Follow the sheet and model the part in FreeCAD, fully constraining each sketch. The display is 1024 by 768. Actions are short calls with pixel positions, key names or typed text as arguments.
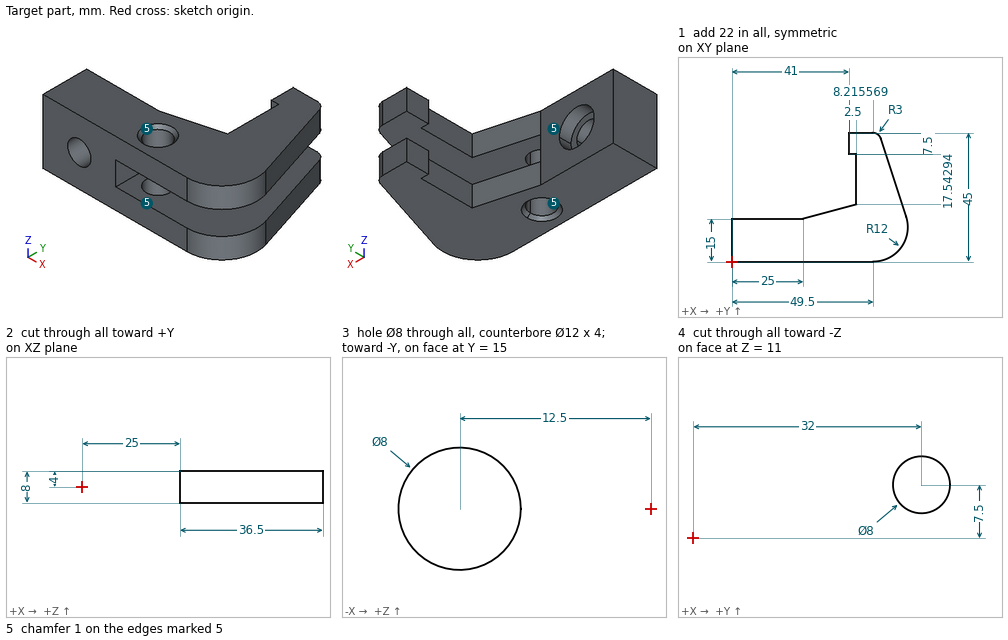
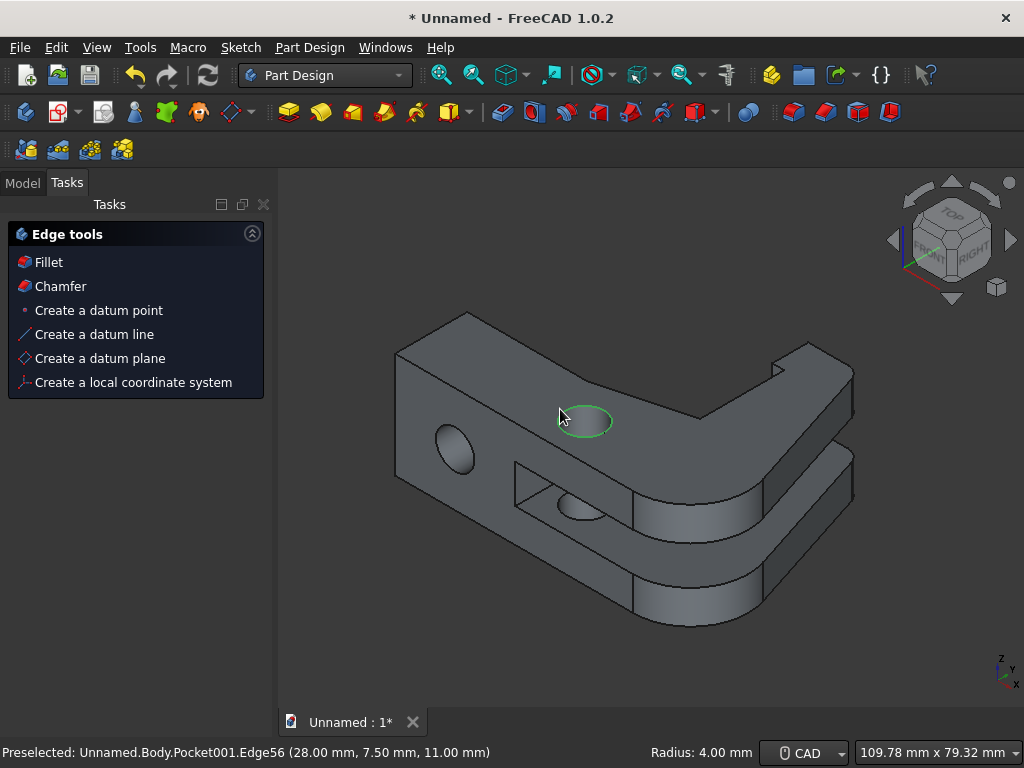
key(2)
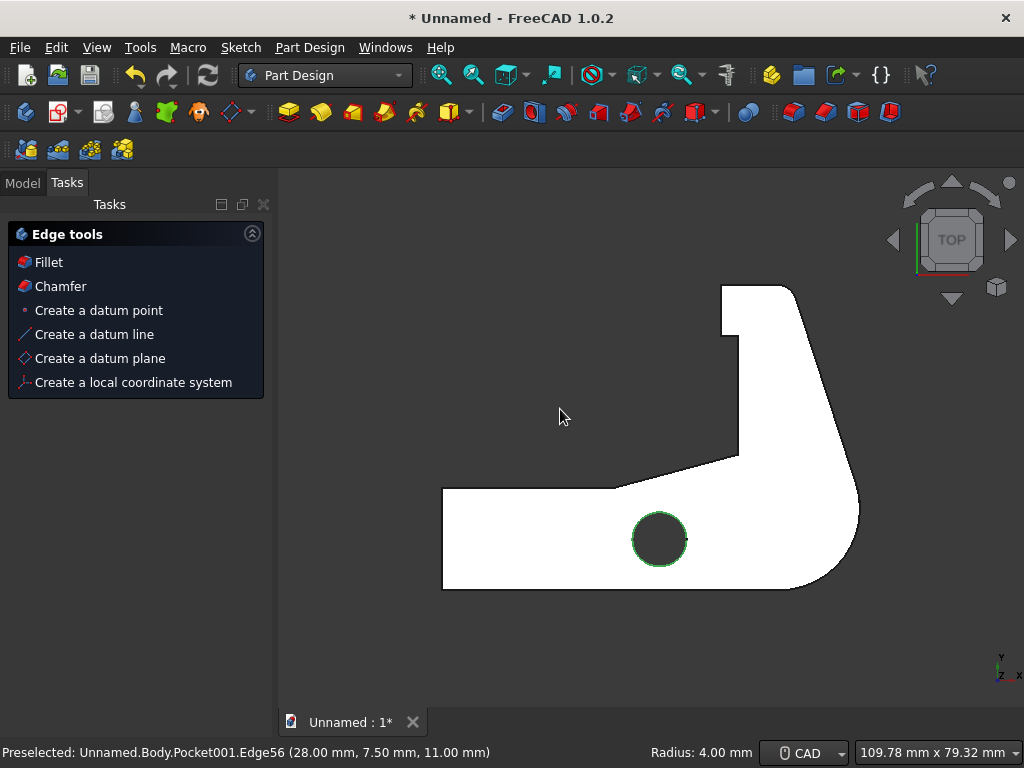
key(0)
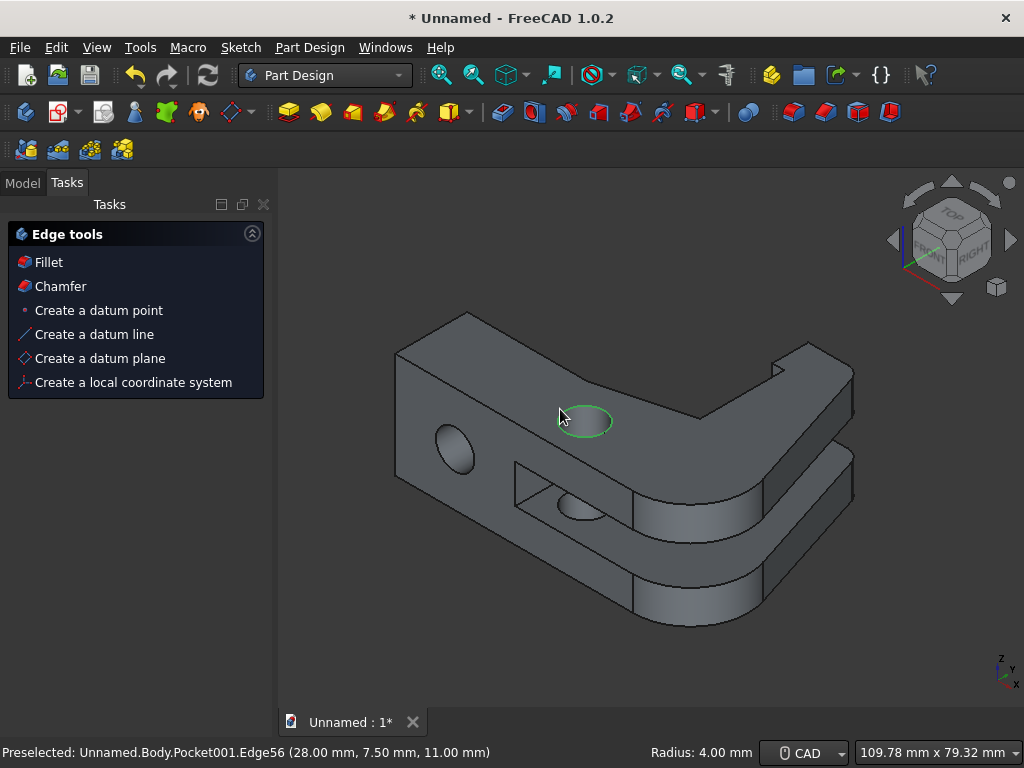
key(1)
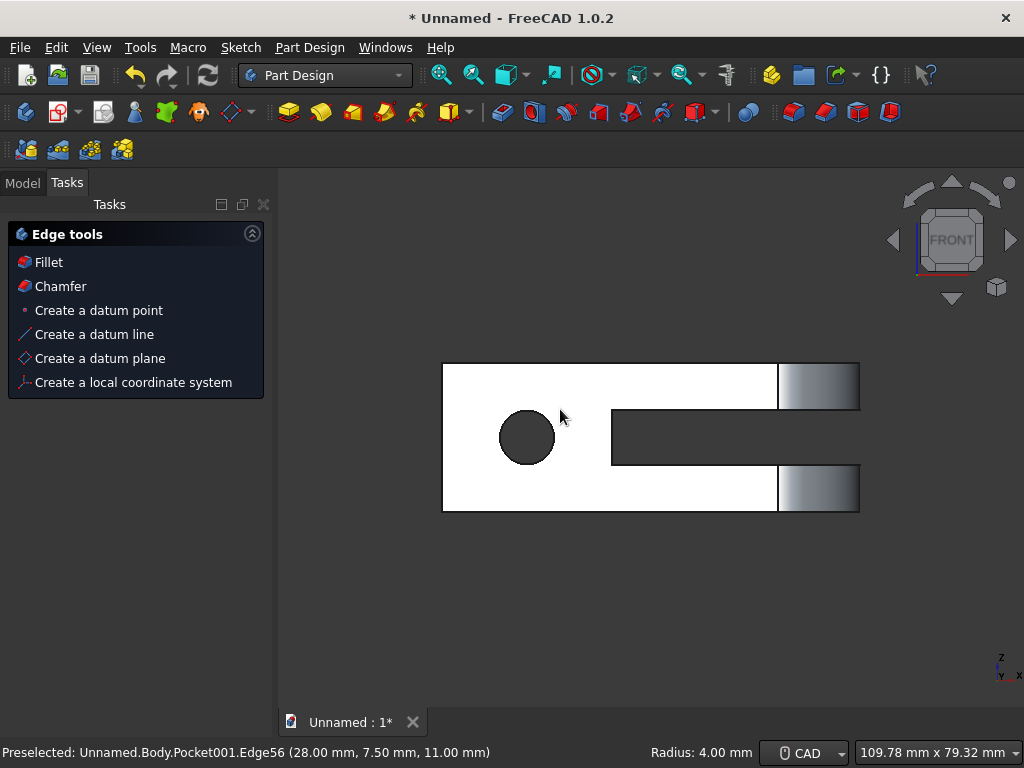
key(3)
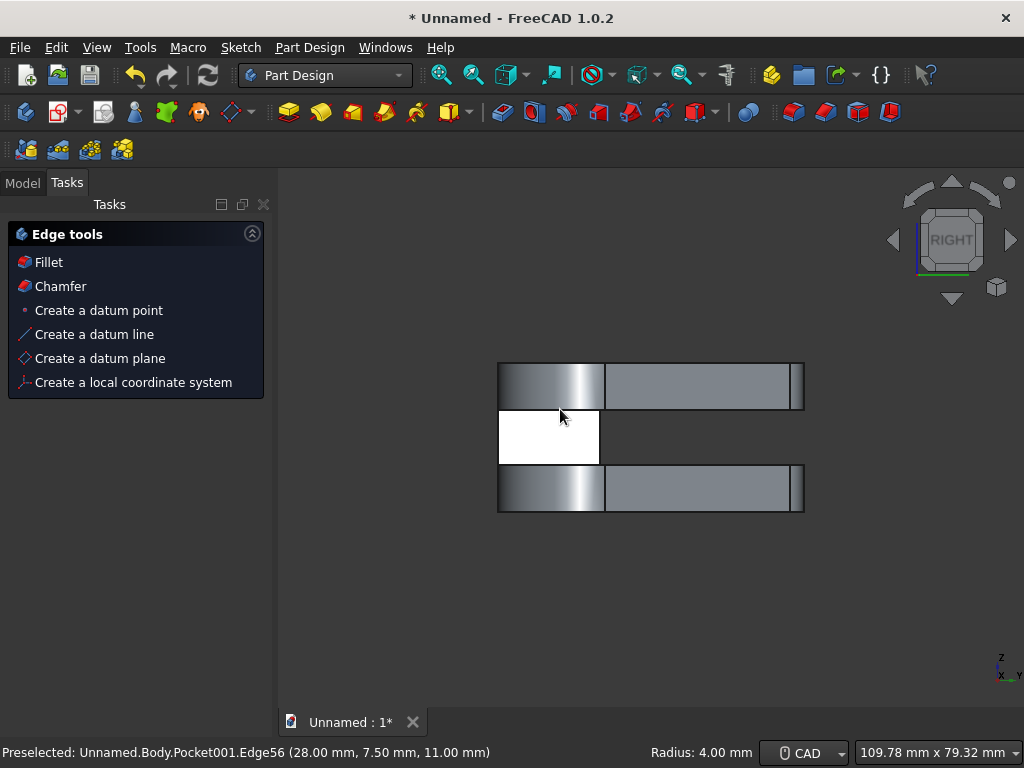
key(v)
key(f)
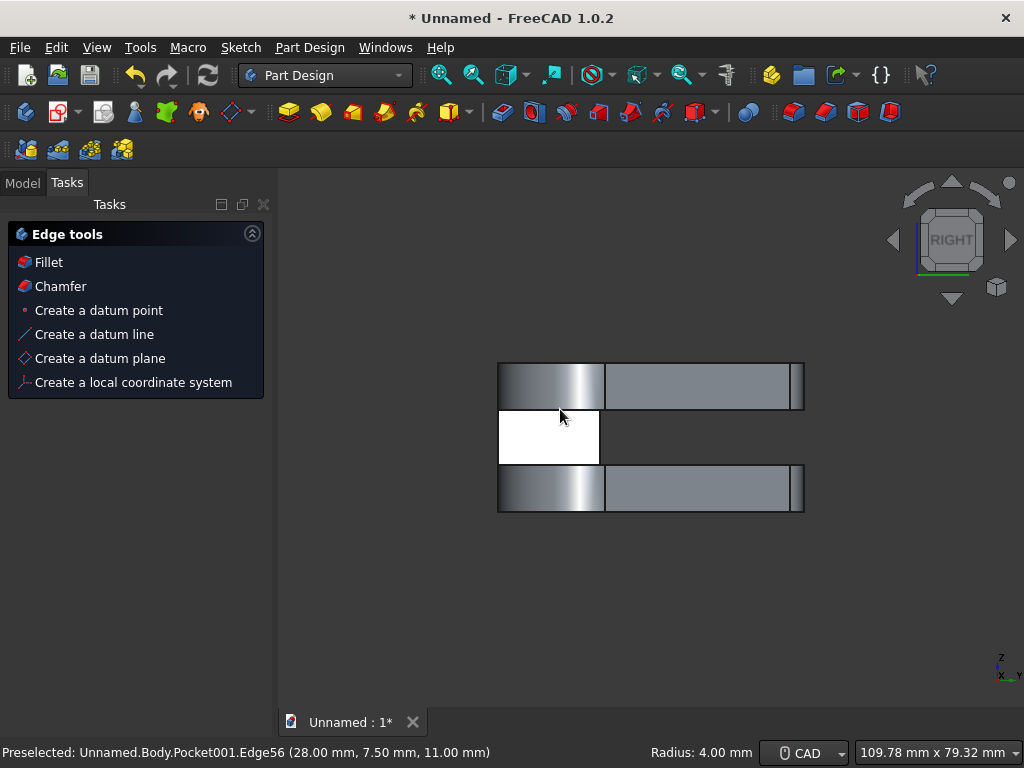
key(5)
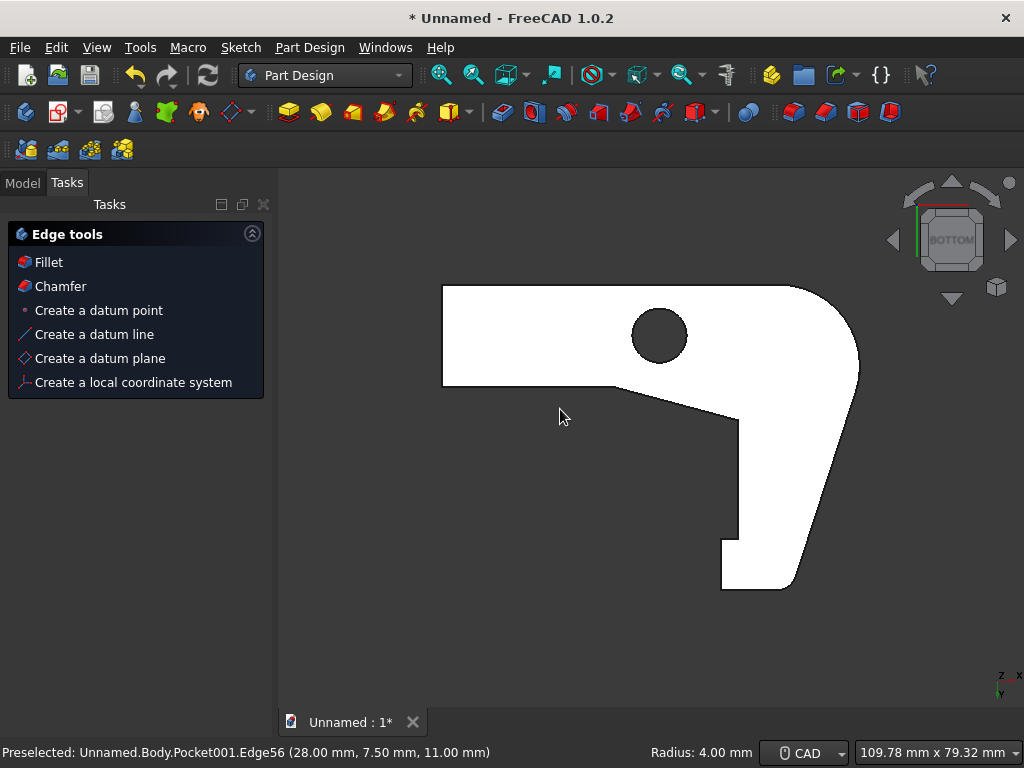
click(632, 335, ctrl)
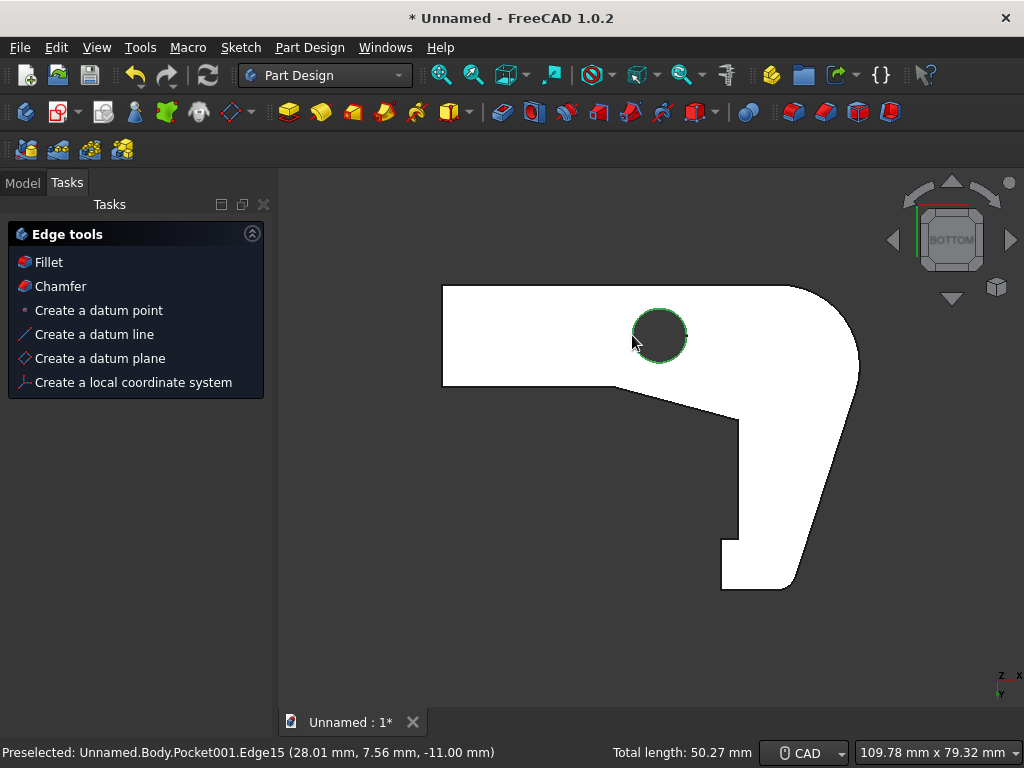
click(826, 112)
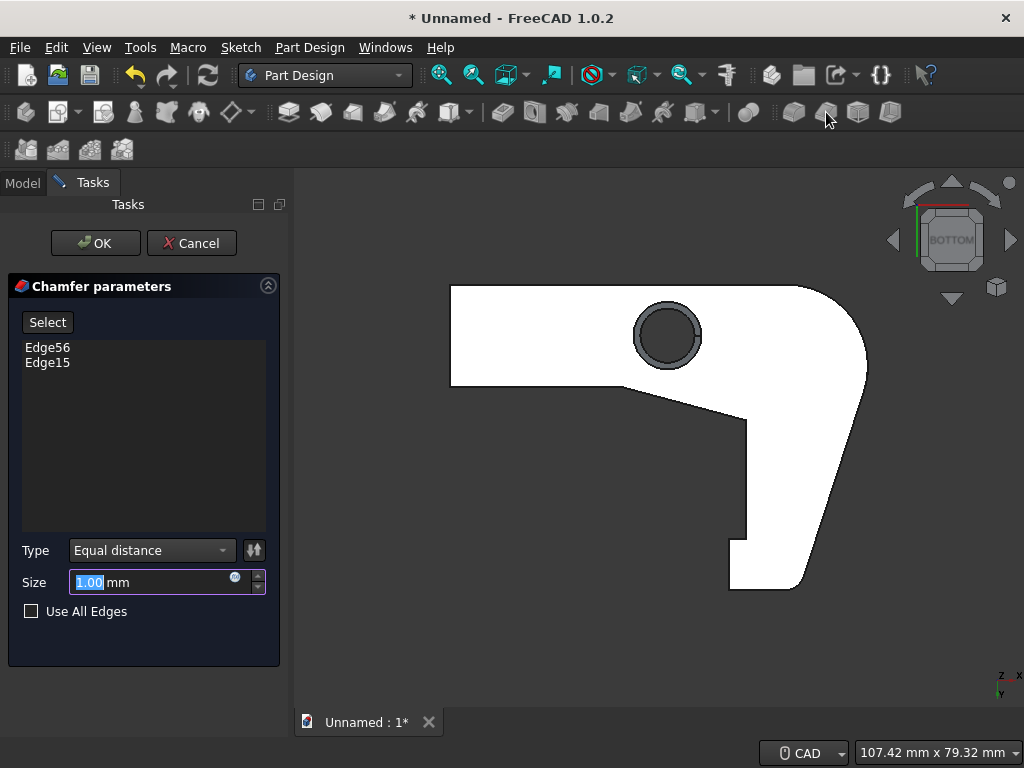
text(1)
key(Tab)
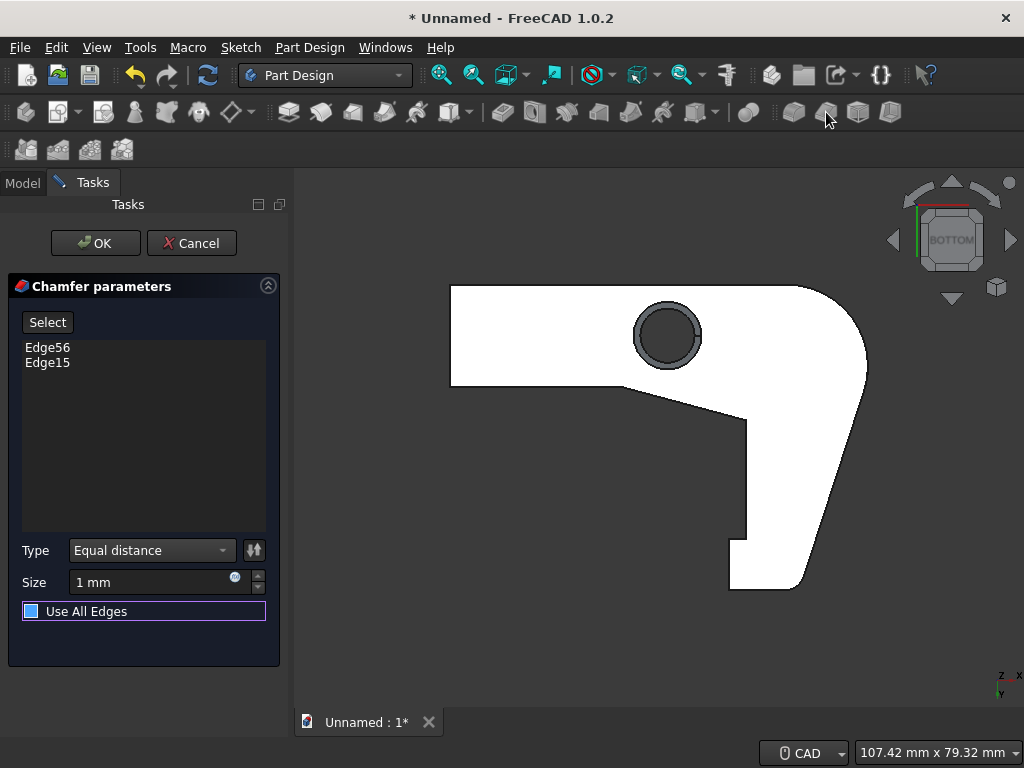
click(96, 243)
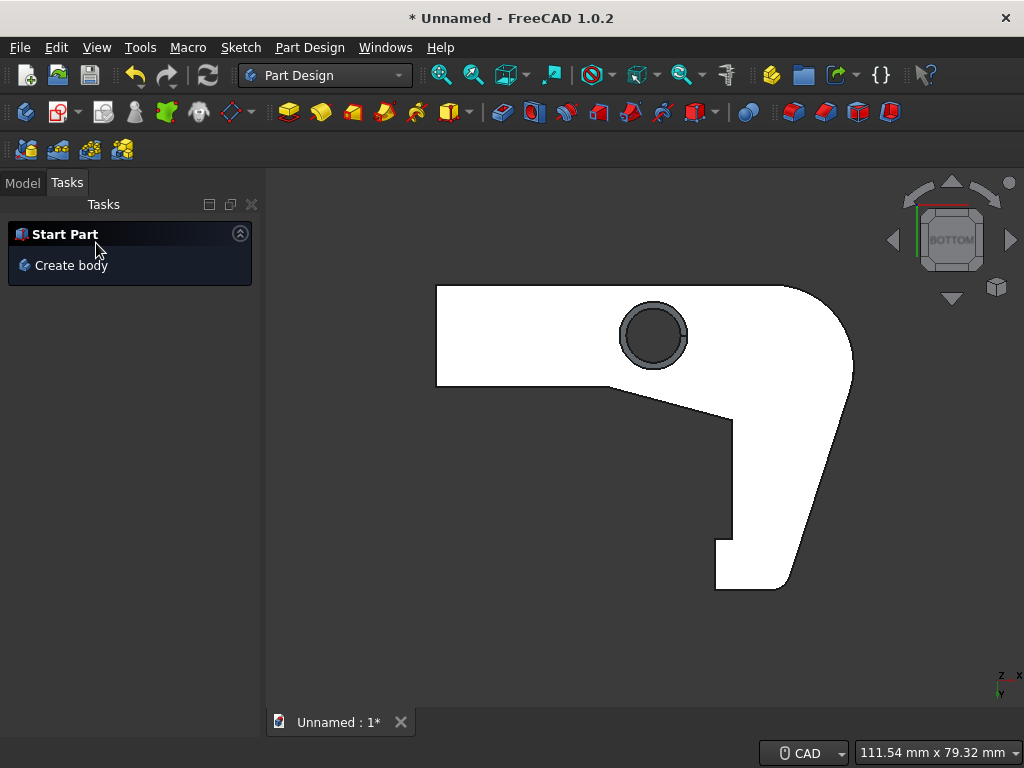
key(0)